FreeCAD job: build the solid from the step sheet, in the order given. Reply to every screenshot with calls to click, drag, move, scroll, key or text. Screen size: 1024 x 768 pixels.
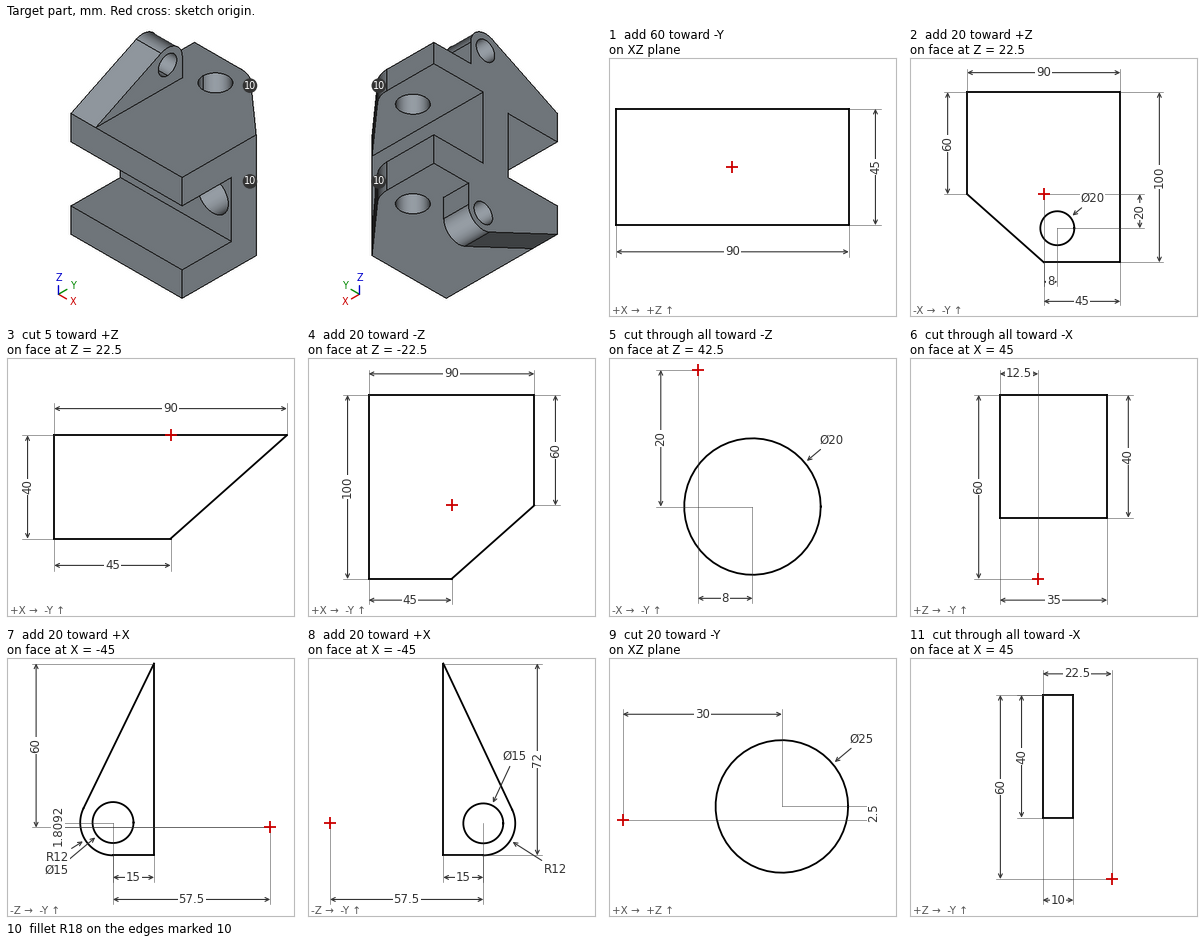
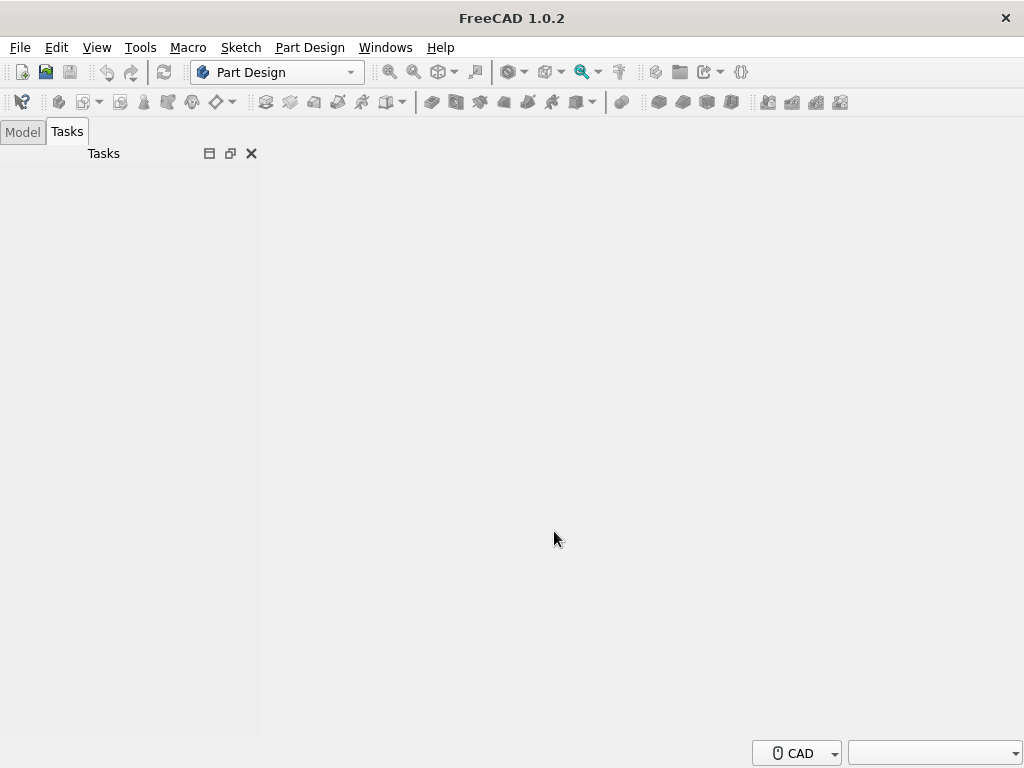
click(22, 72)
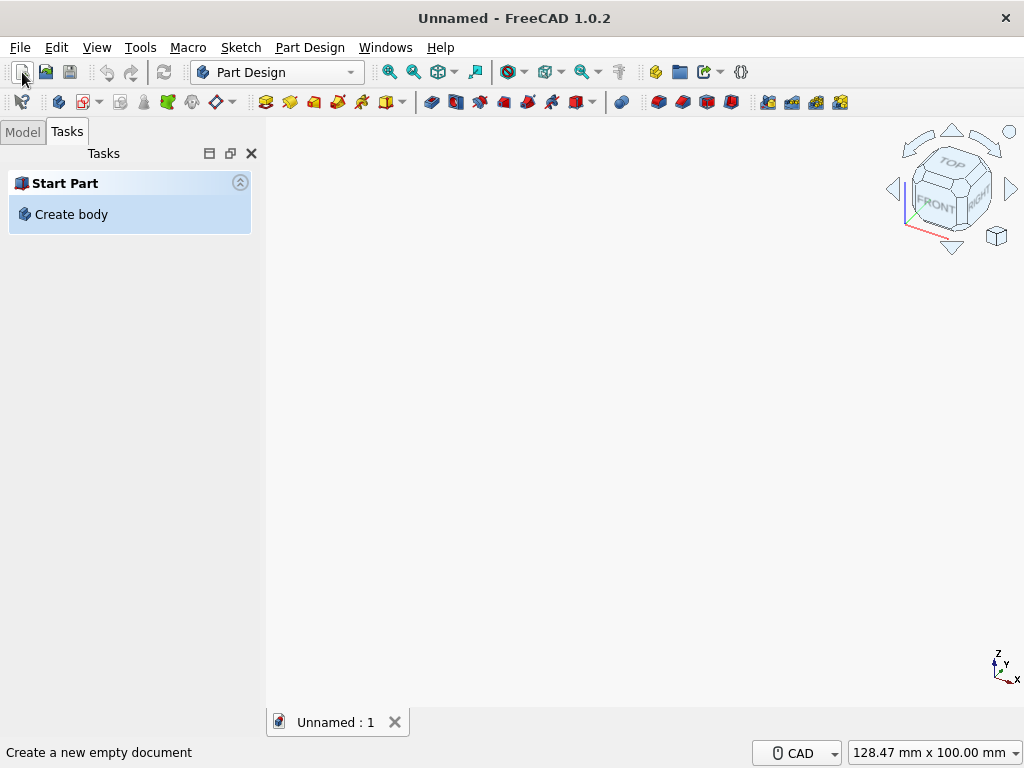
click(84, 102)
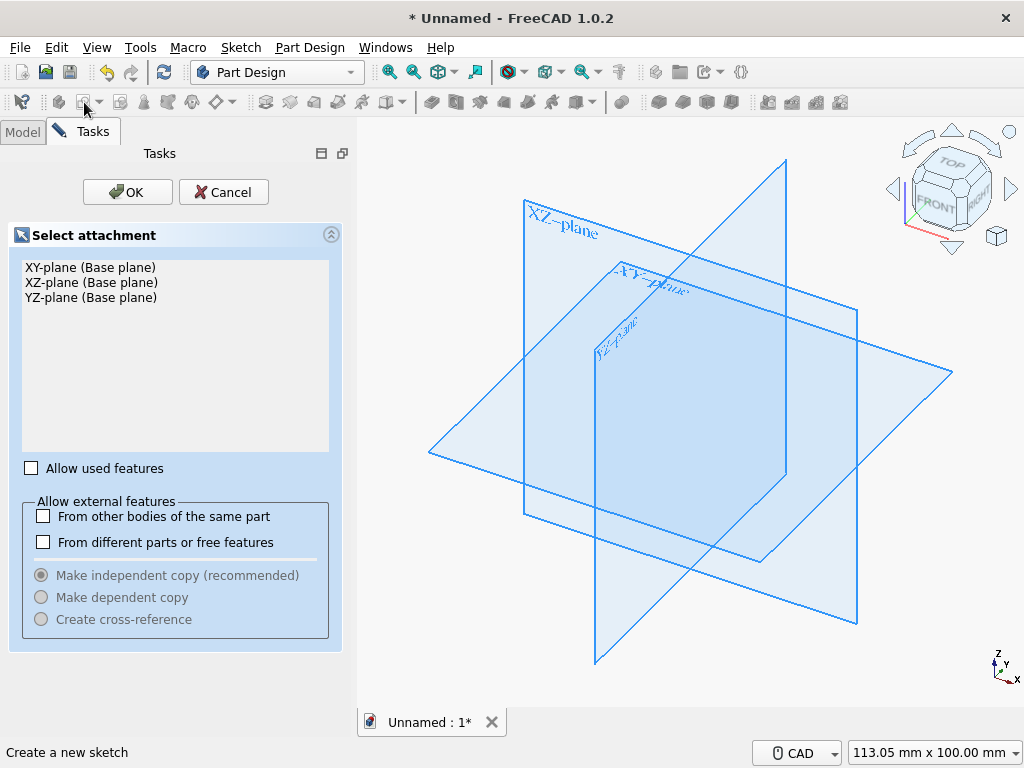
click(82, 282)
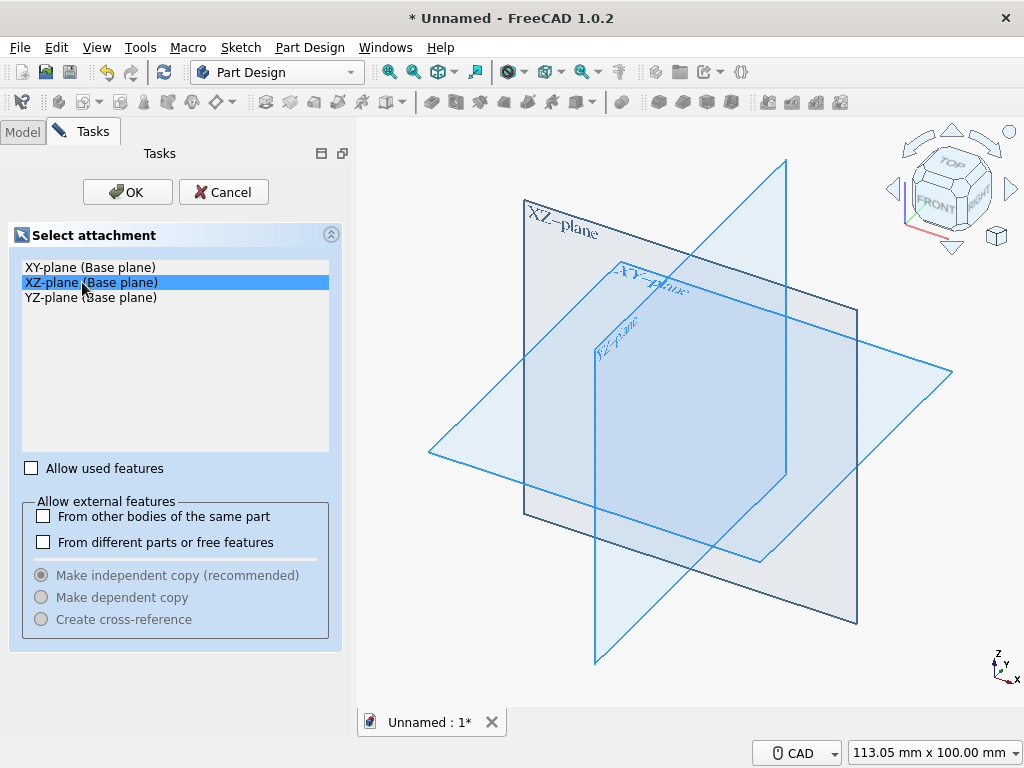
click(128, 192)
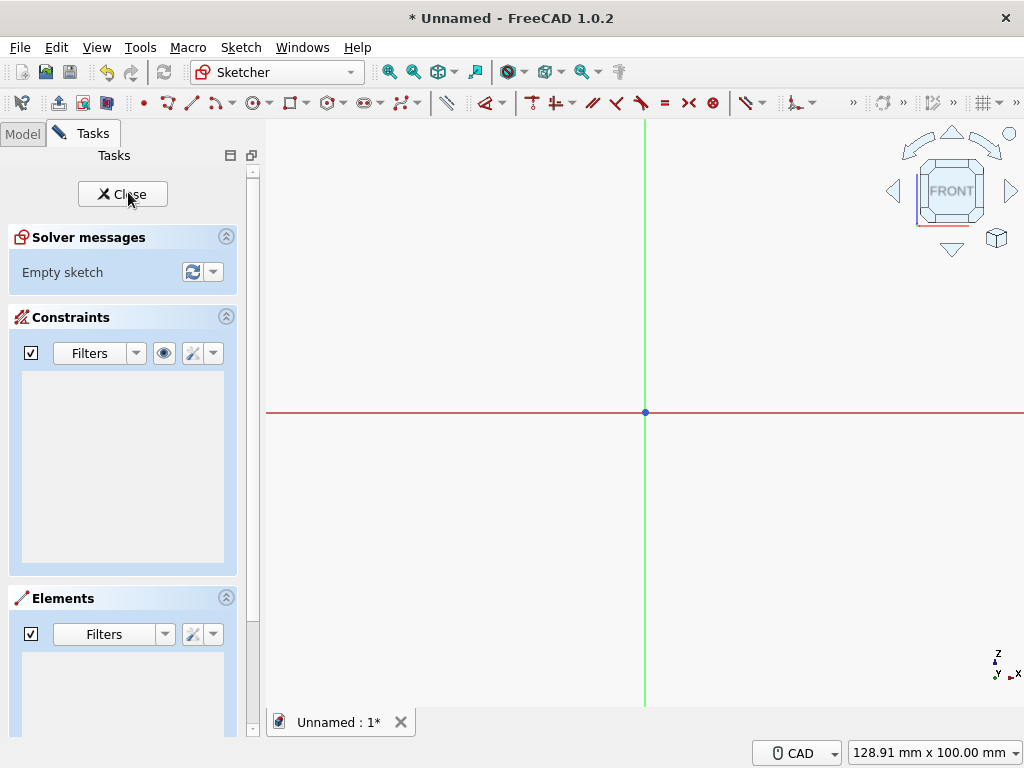
scroll(294, 413, down, 1)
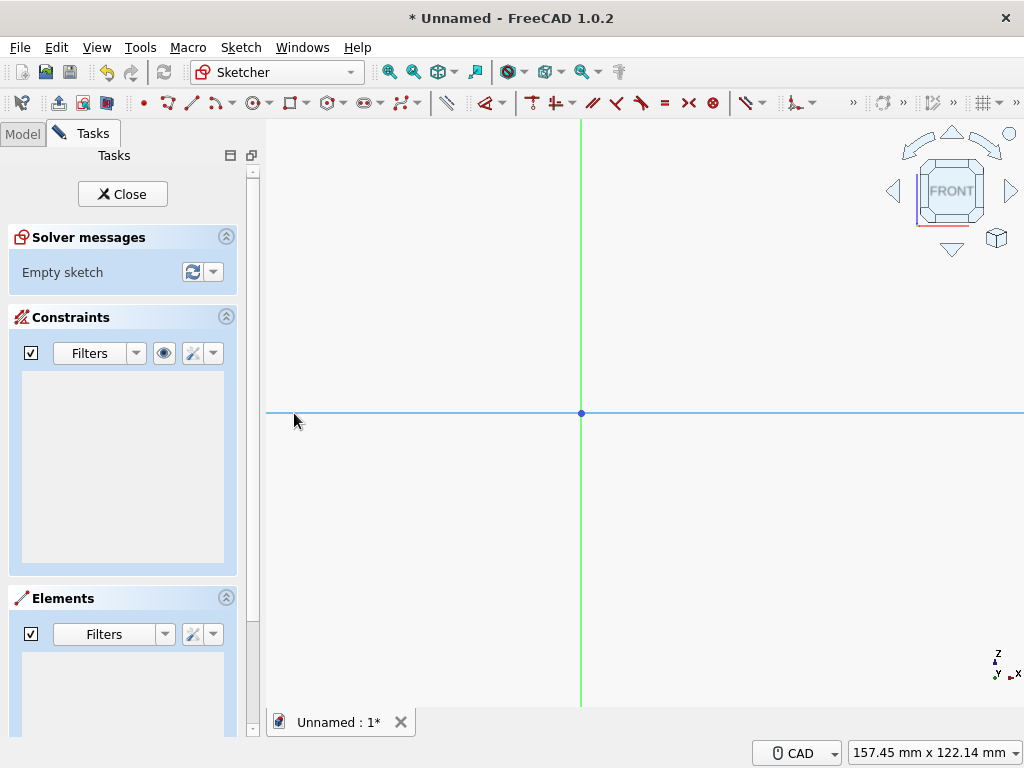
key(g)
key(v)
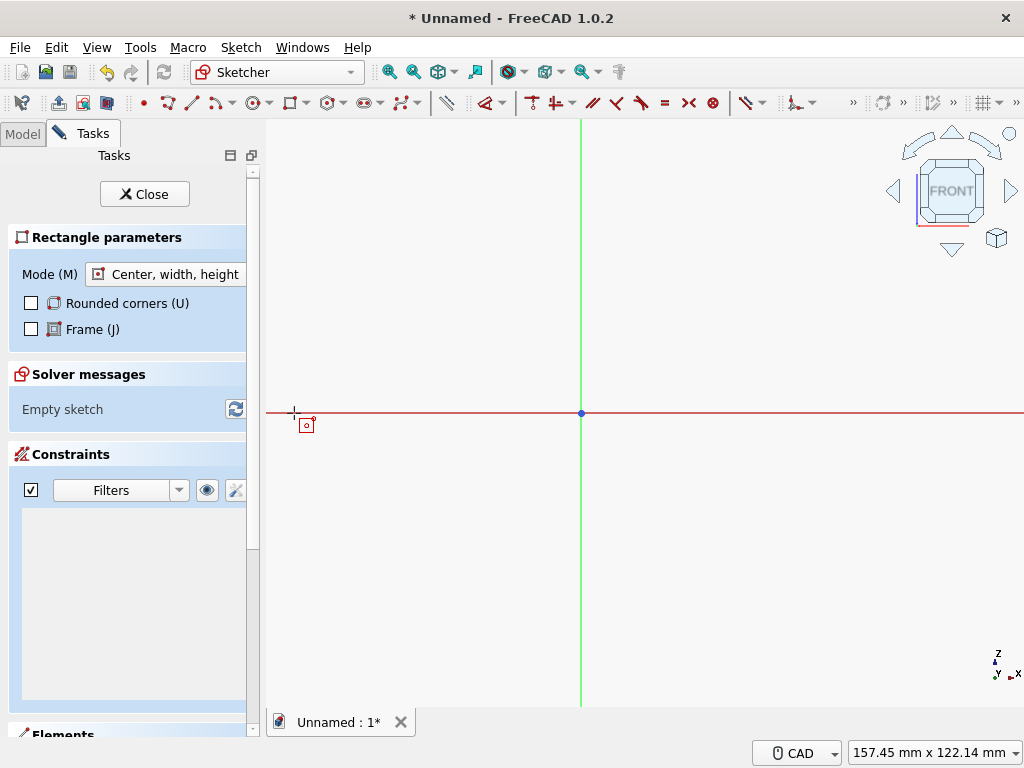
click(581, 413)
move(798, 305)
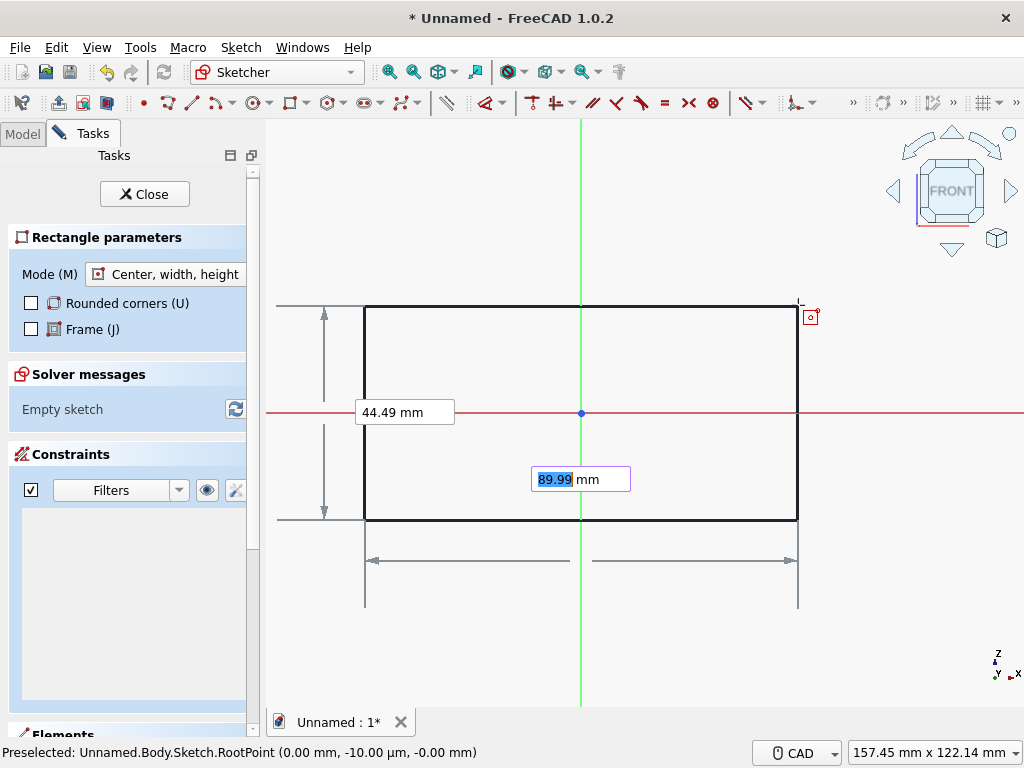
text(90)
key(Tab)
text(45)
key(Return)
key(Escape)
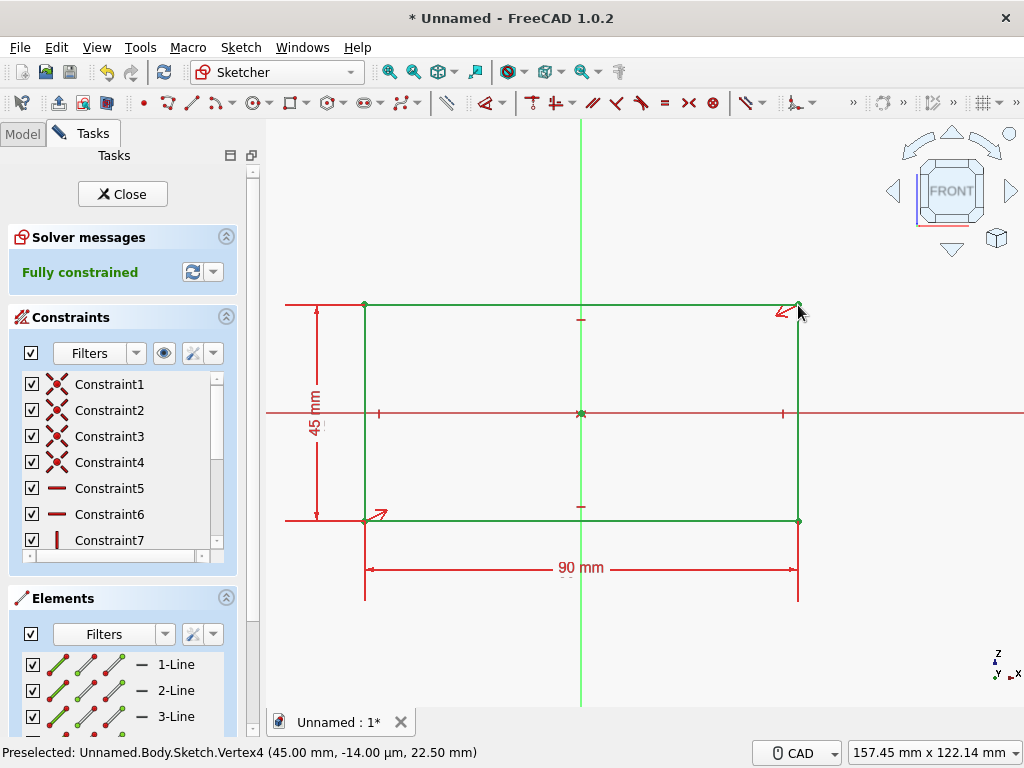
click(123, 194)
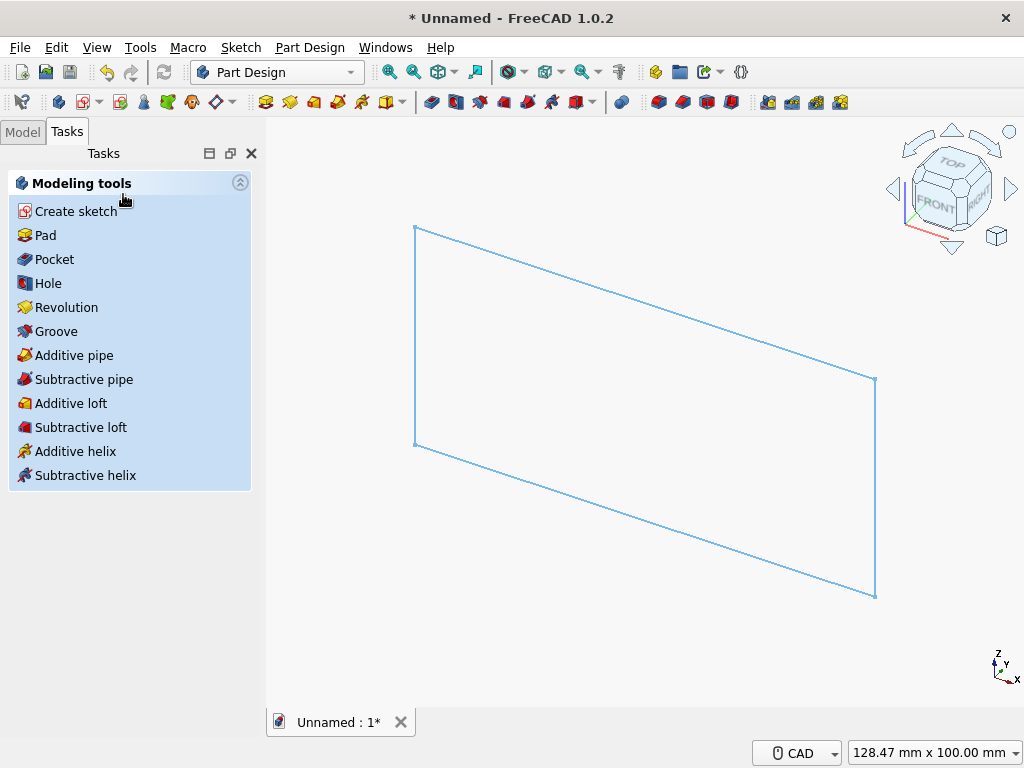
click(266, 102)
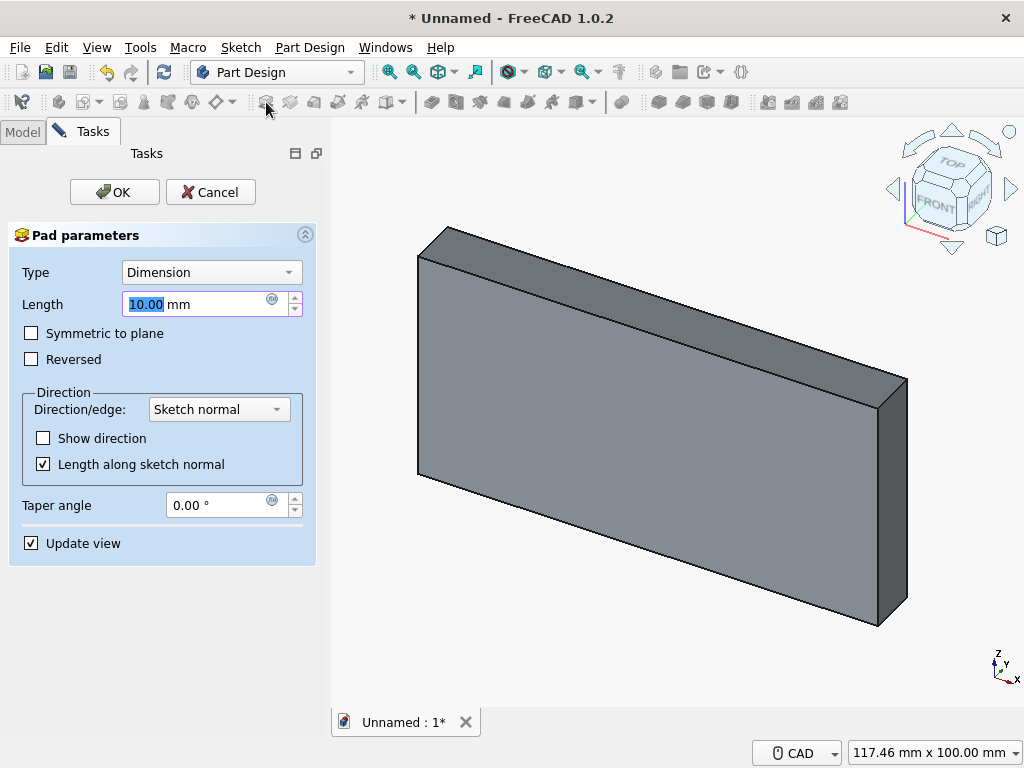
text(60)
key(Tab)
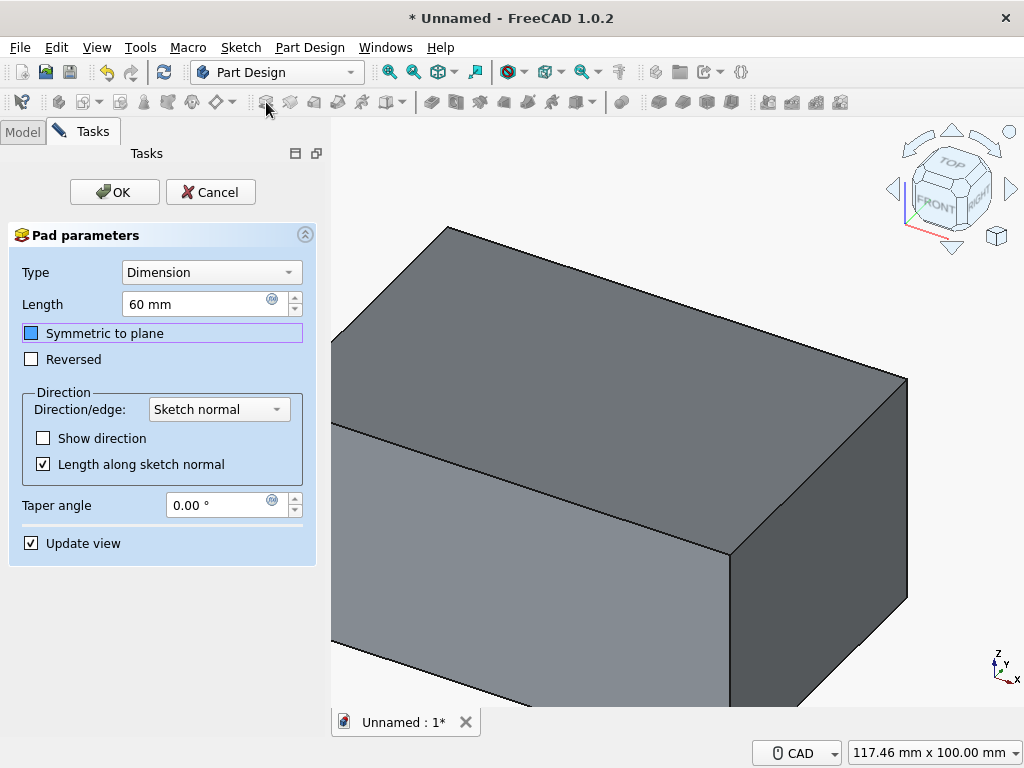
click(115, 192)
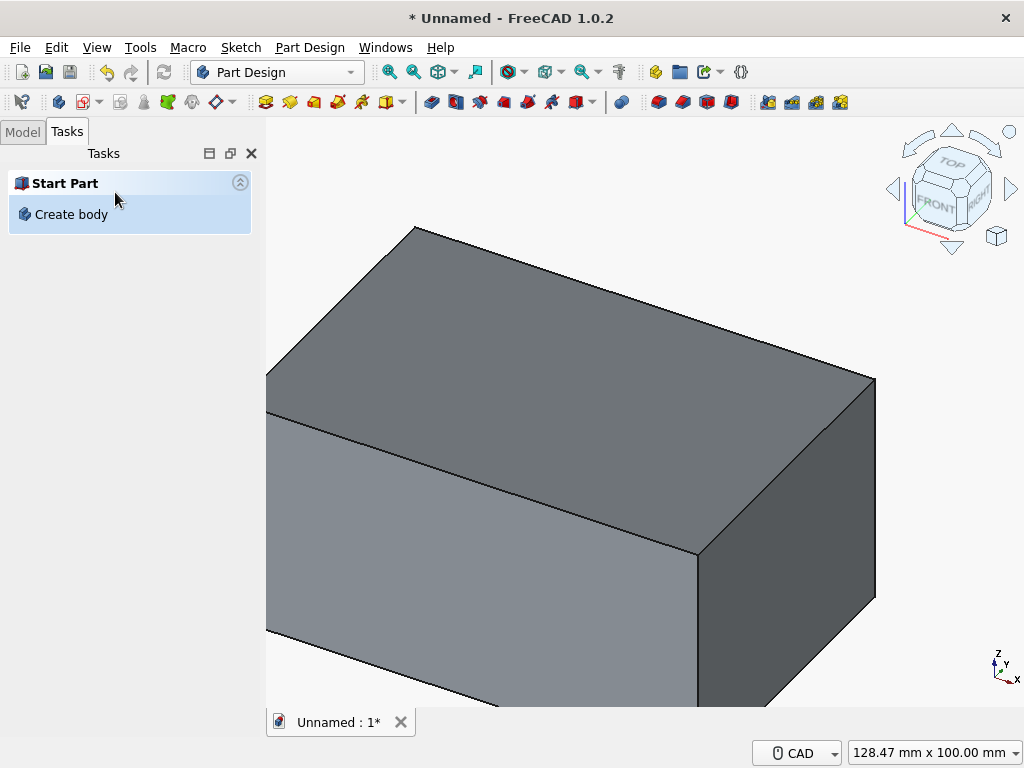
key(v)
key(f)